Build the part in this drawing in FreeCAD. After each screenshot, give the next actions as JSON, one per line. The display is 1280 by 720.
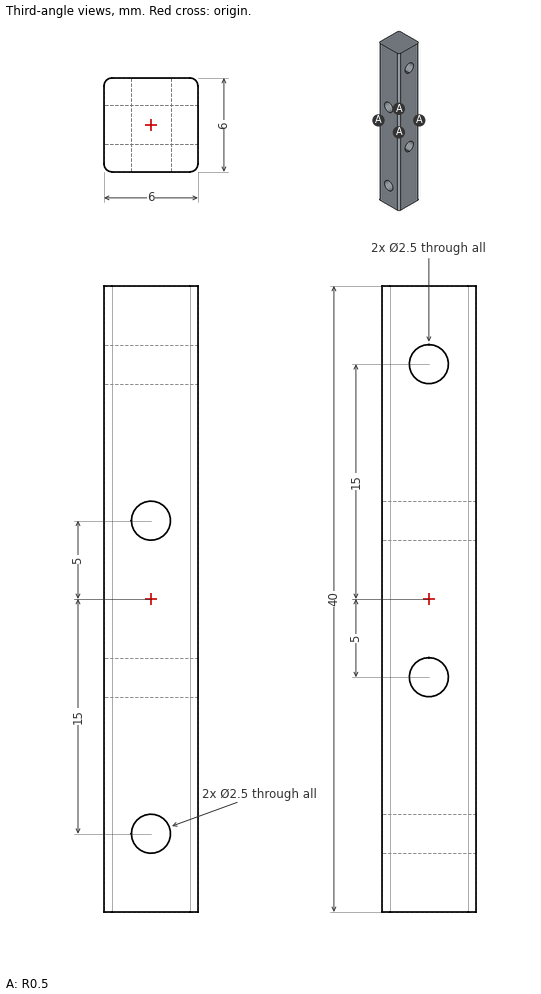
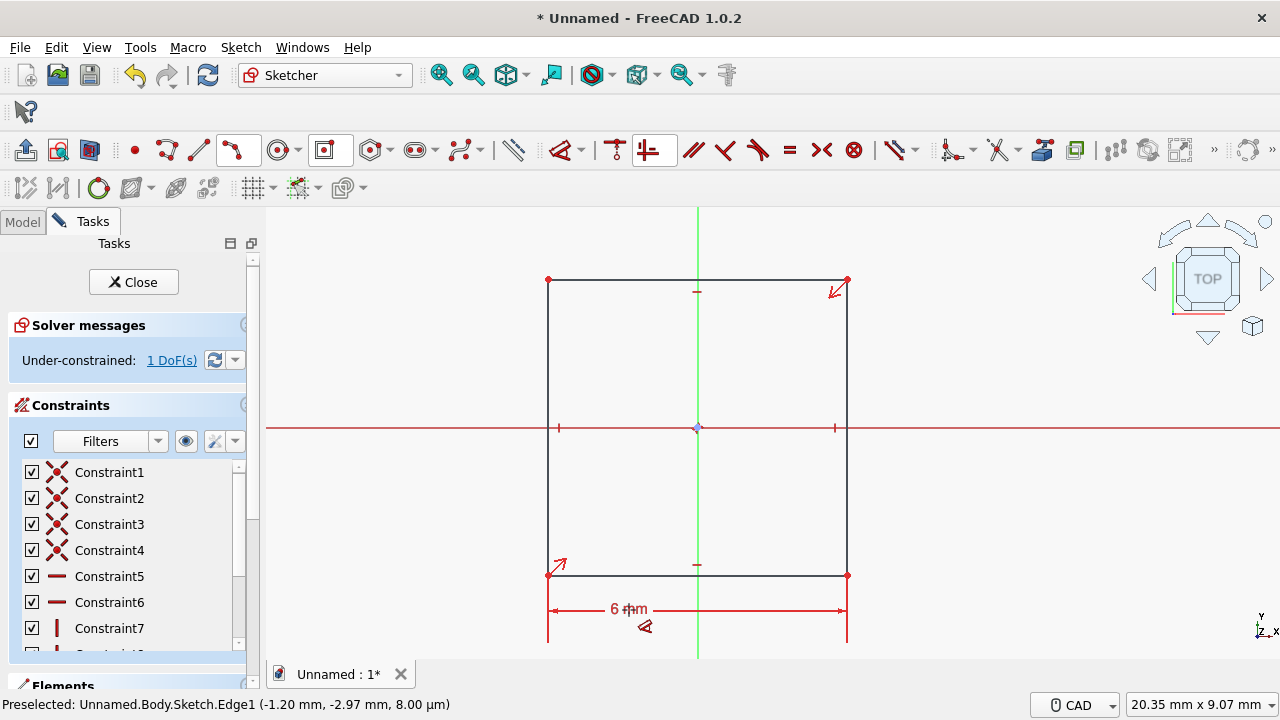
{"action": "left_click", "coordinate": [847, 487]}
{"action": "left_click", "coordinate": [881, 360]}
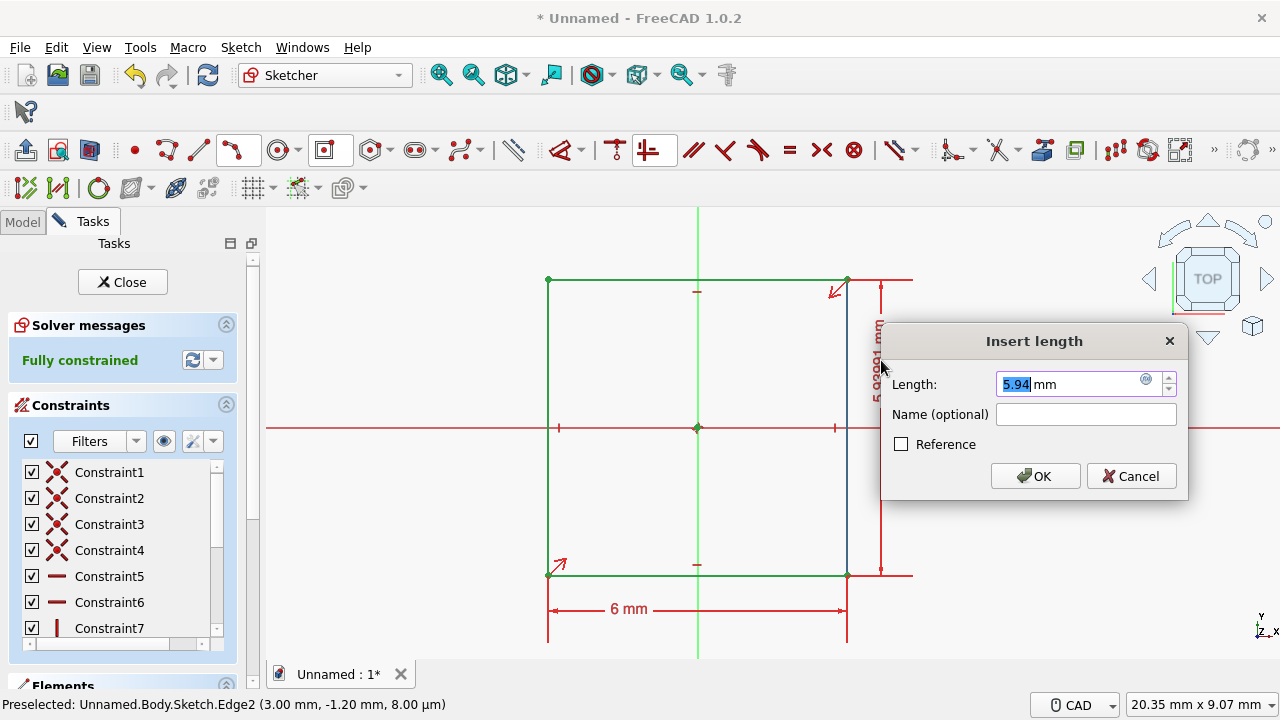
{"action": "type", "text": "6"}
{"action": "key", "text": "Return"}
{"action": "key", "text": "Escape"}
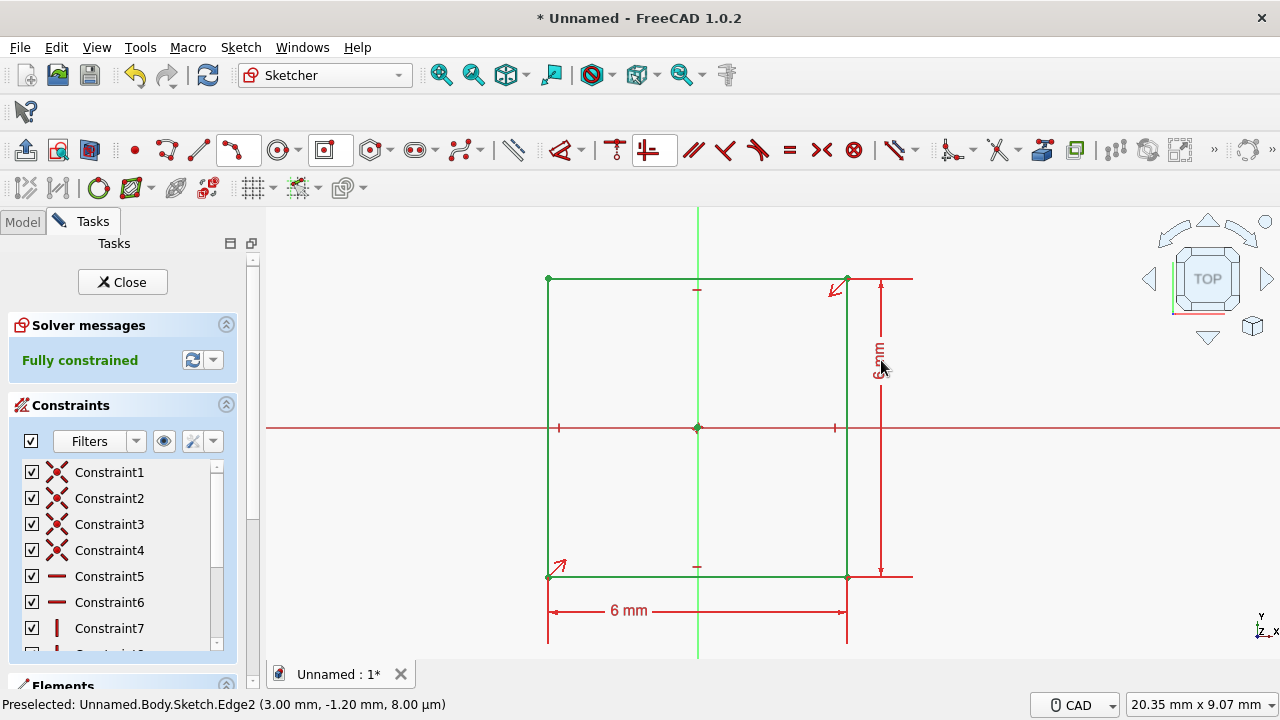
{"action": "left_click", "coordinate": [123, 282]}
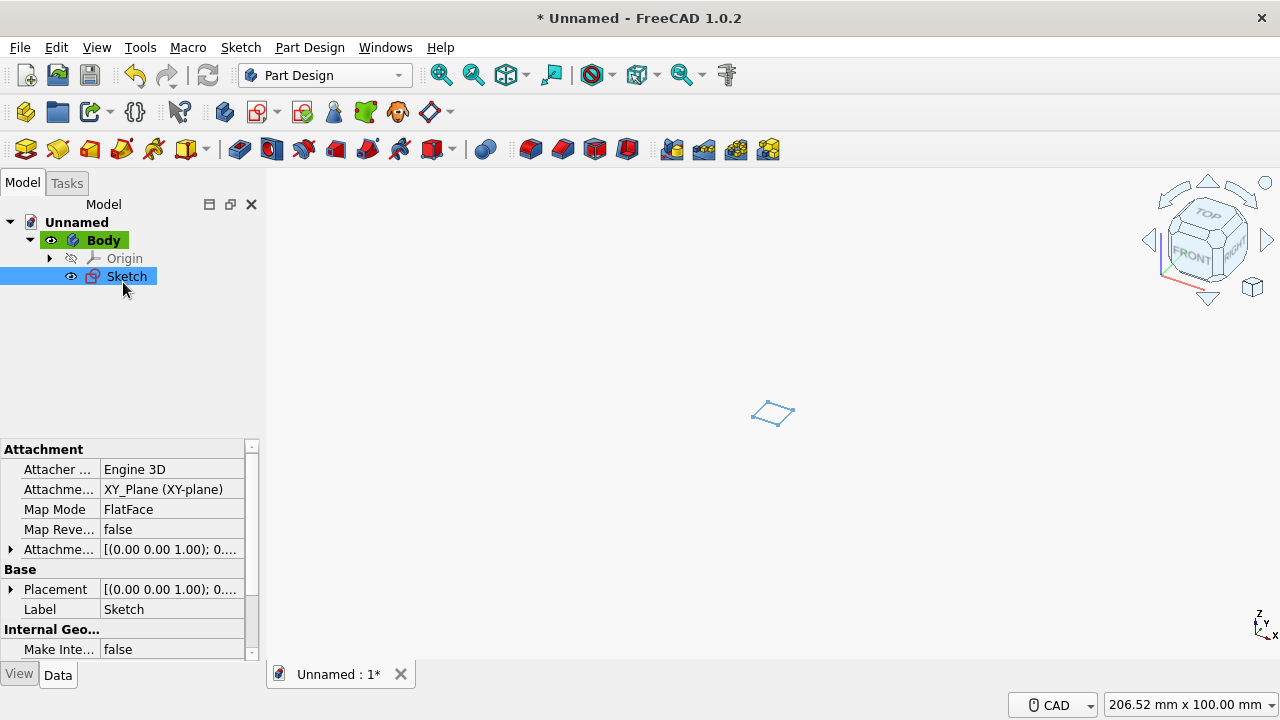
{"action": "left_click", "coordinate": [26, 150]}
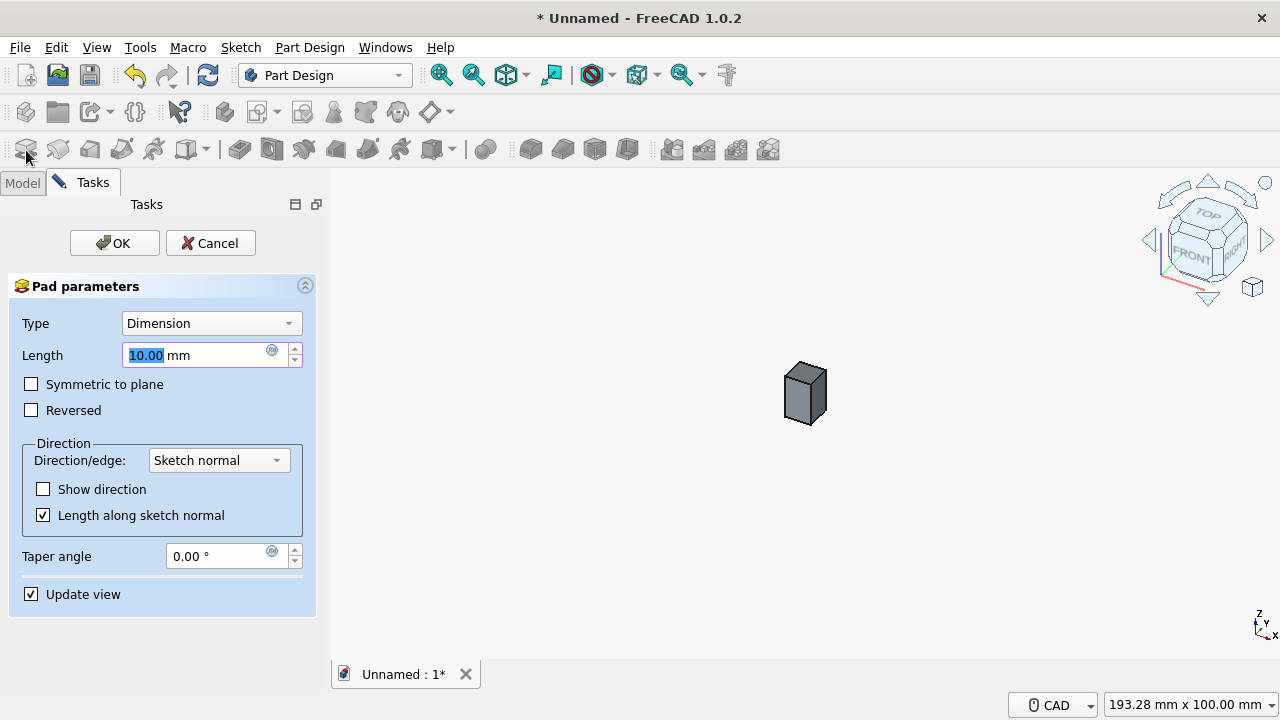
{"action": "type", "text": "40"}
{"action": "key", "text": "Tab"}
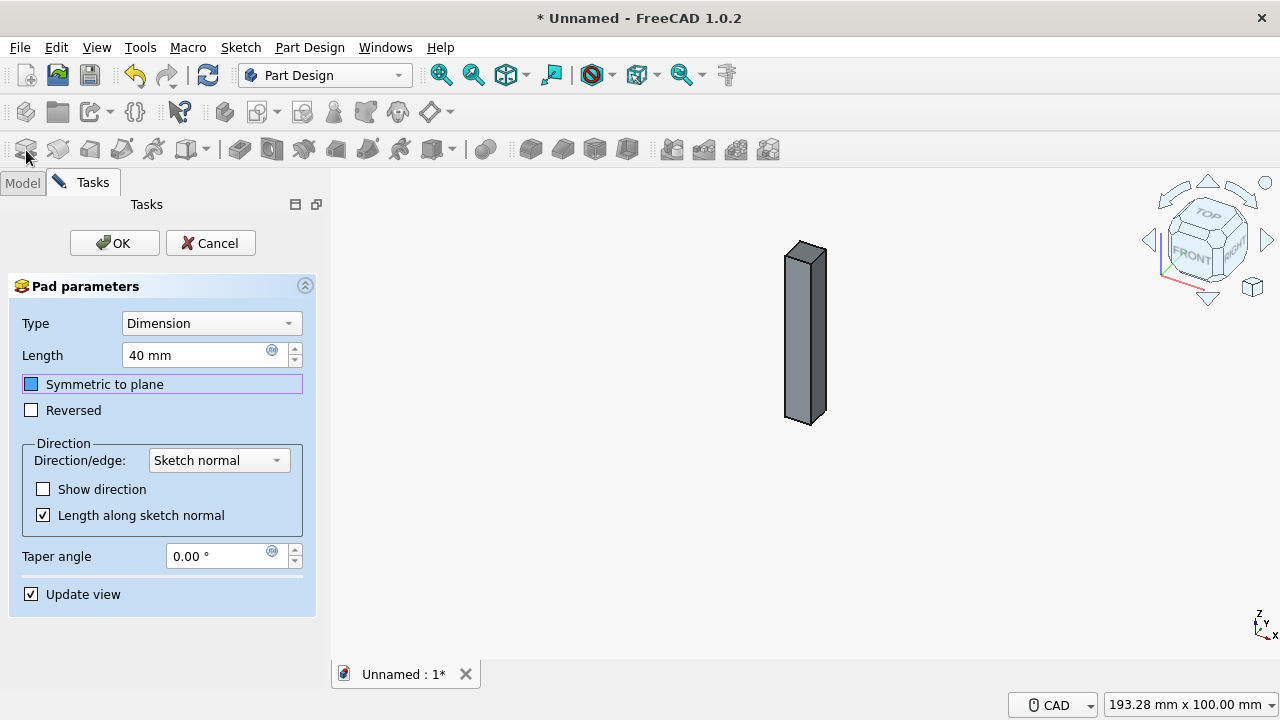
{"action": "left_click", "coordinate": [30, 384]}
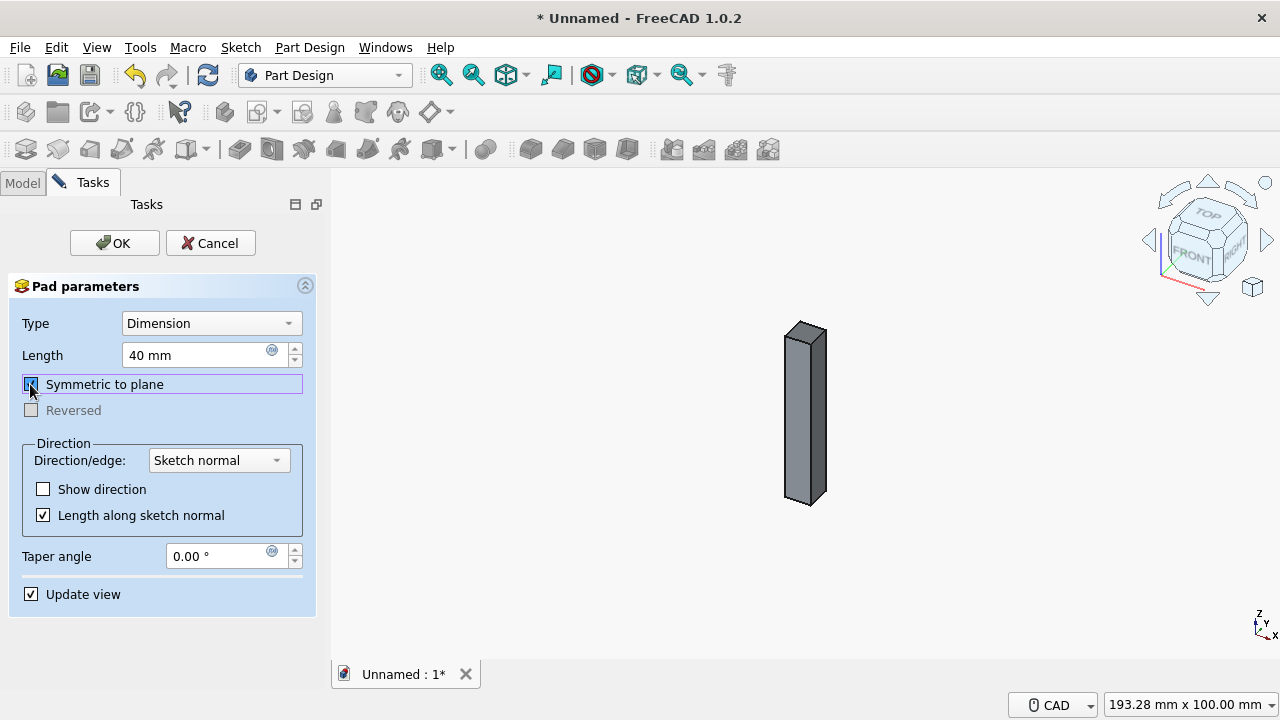
{"action": "left_click", "coordinate": [115, 243]}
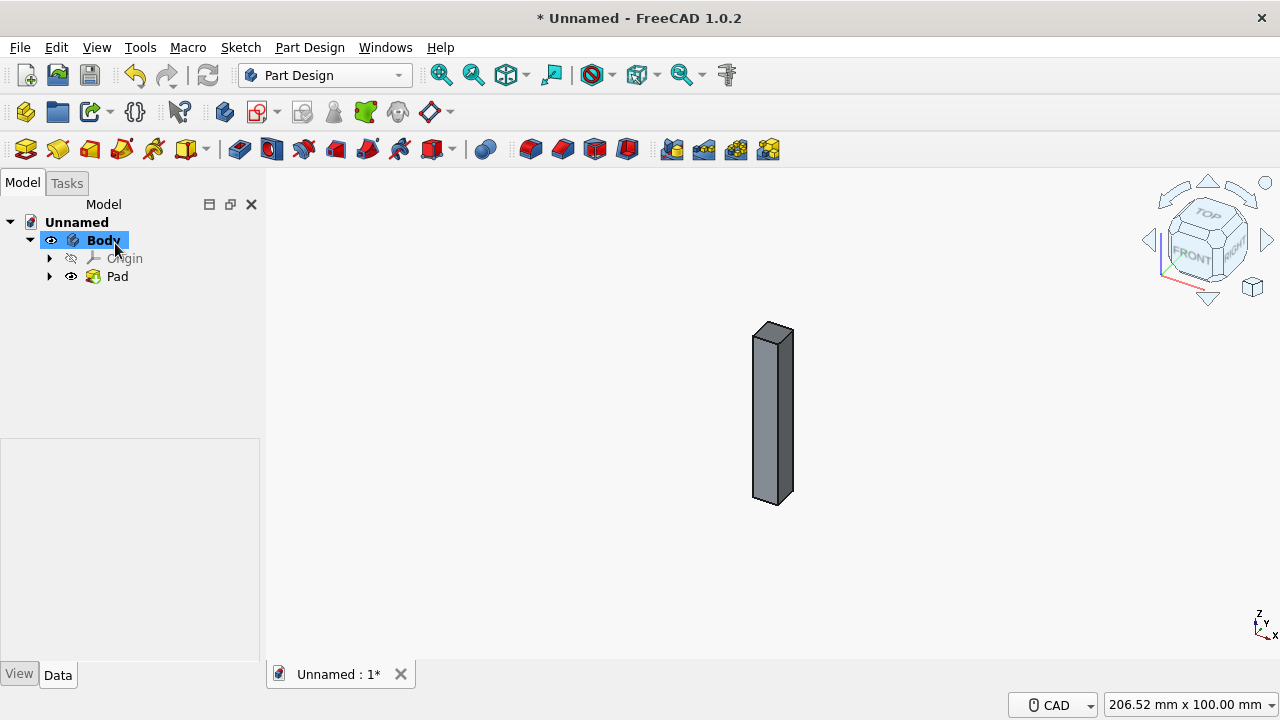
{"action": "left_click", "coordinate": [442, 76]}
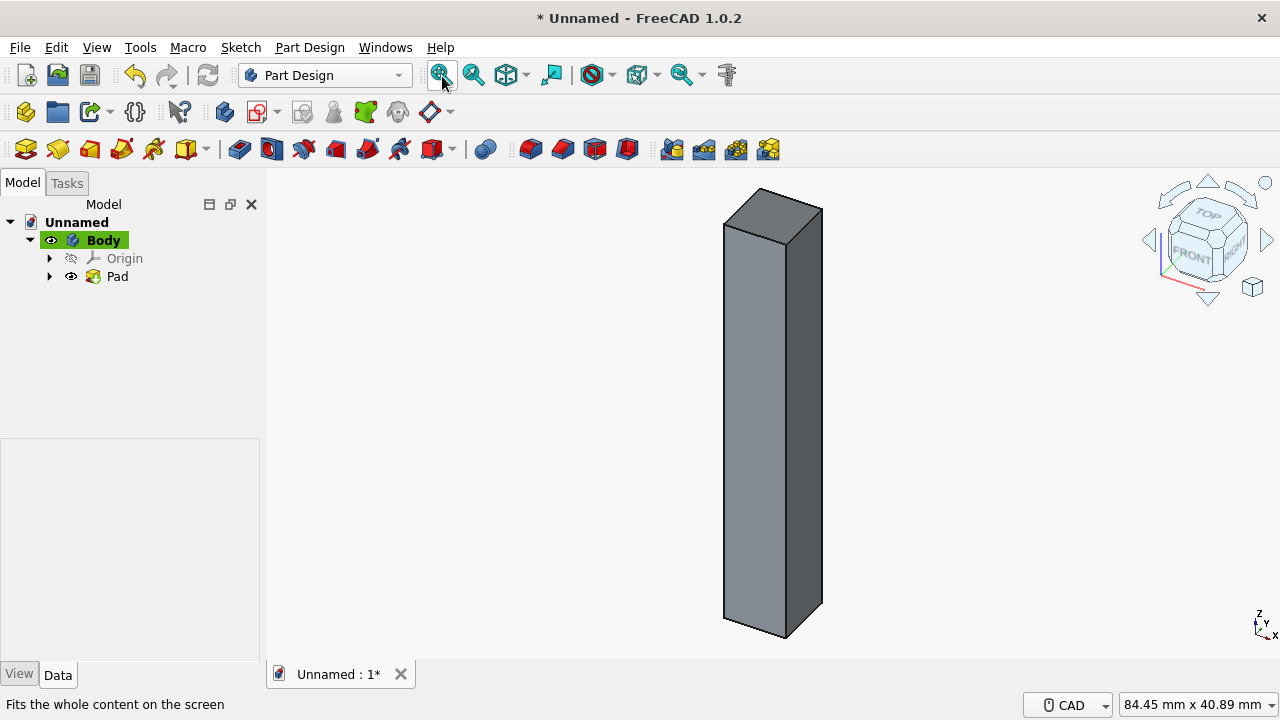
{"action": "key", "text": "4"}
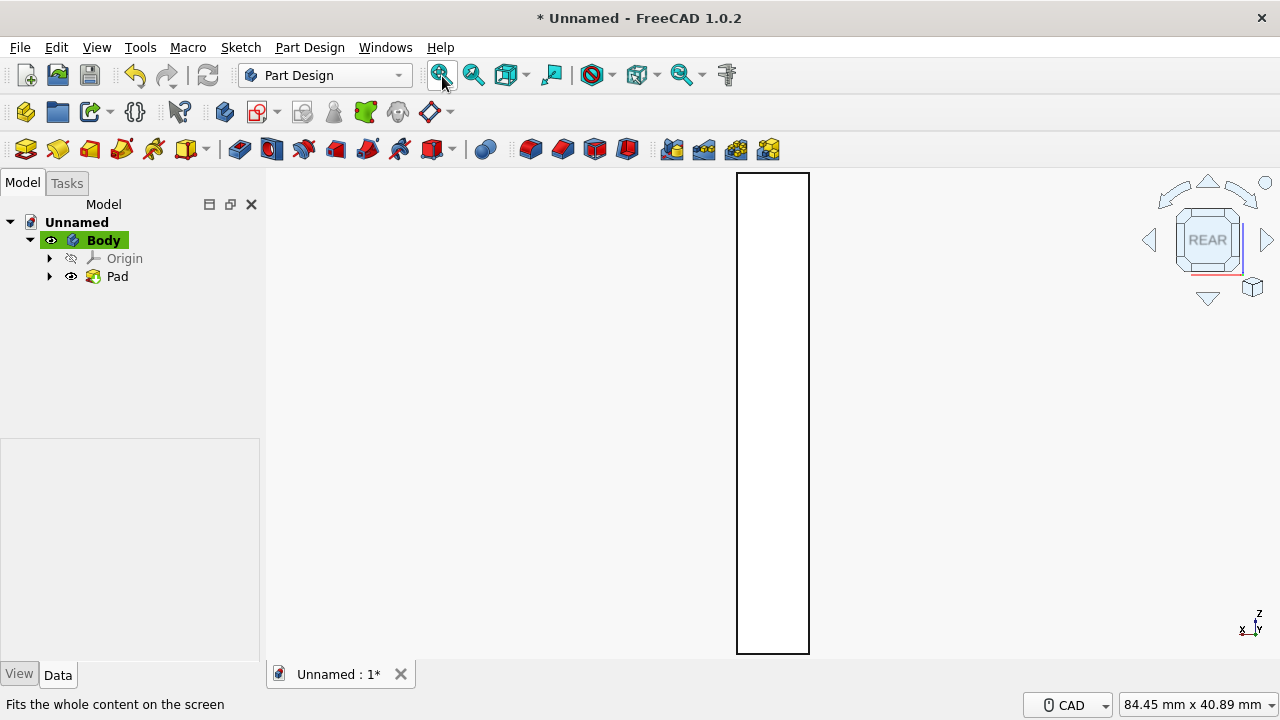
{"action": "left_click", "coordinate": [773, 275]}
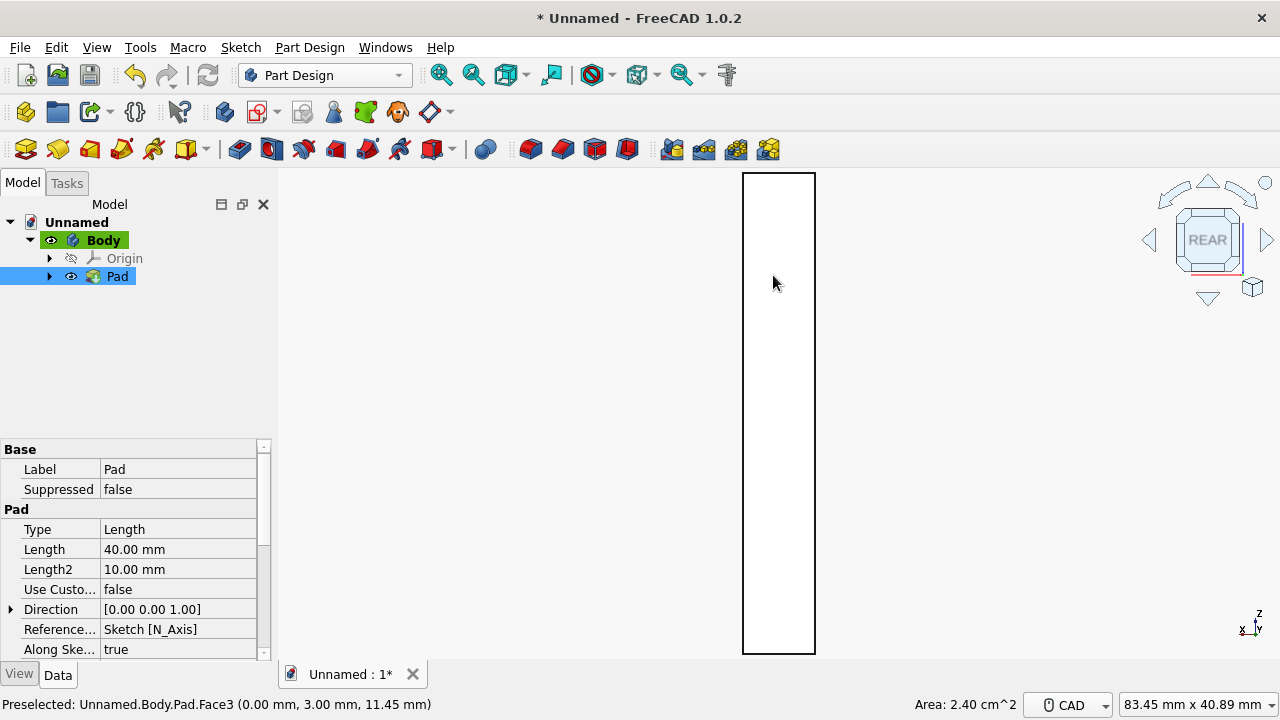
{"action": "left_click", "coordinate": [258, 112]}